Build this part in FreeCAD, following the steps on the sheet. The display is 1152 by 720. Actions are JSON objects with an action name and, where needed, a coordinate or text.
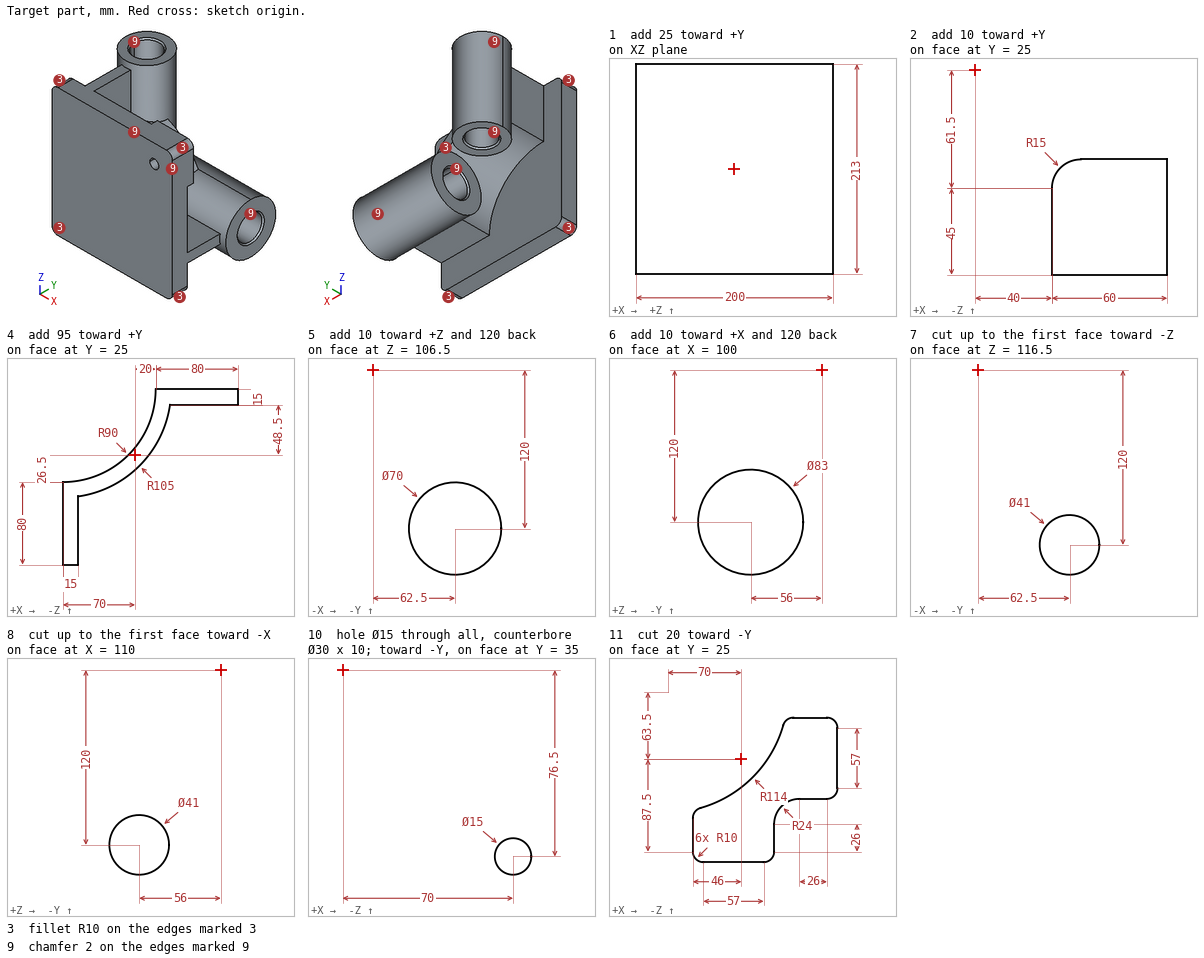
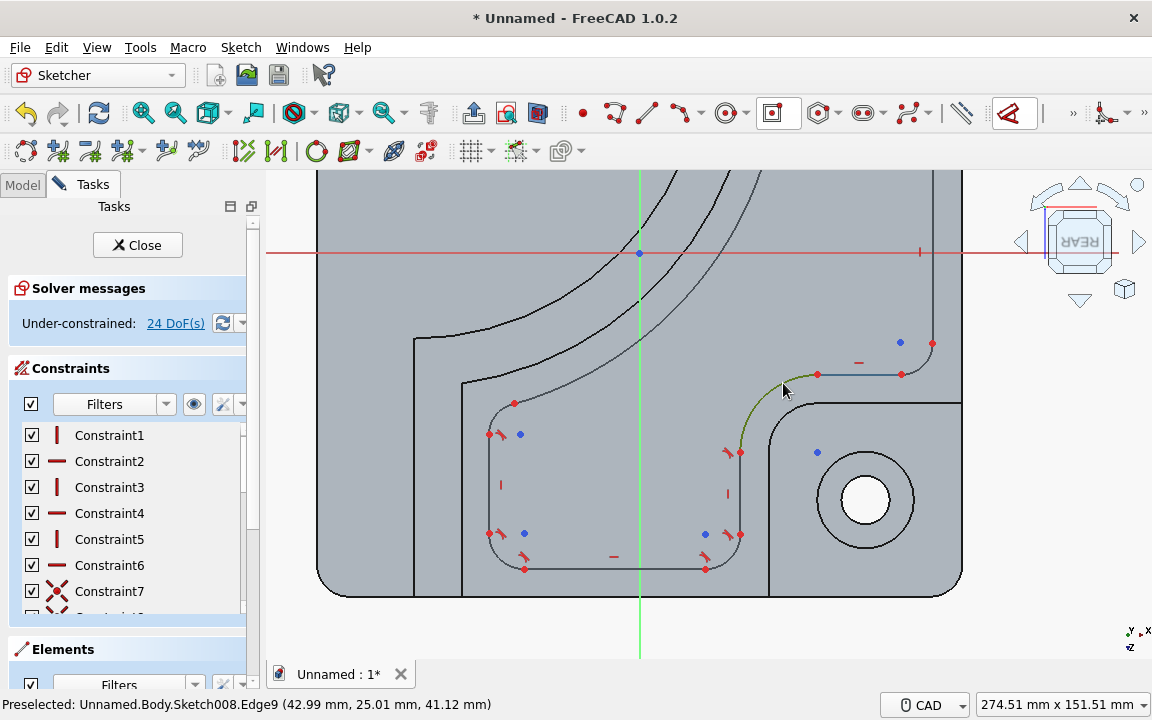
{"action": "key", "text": "t"}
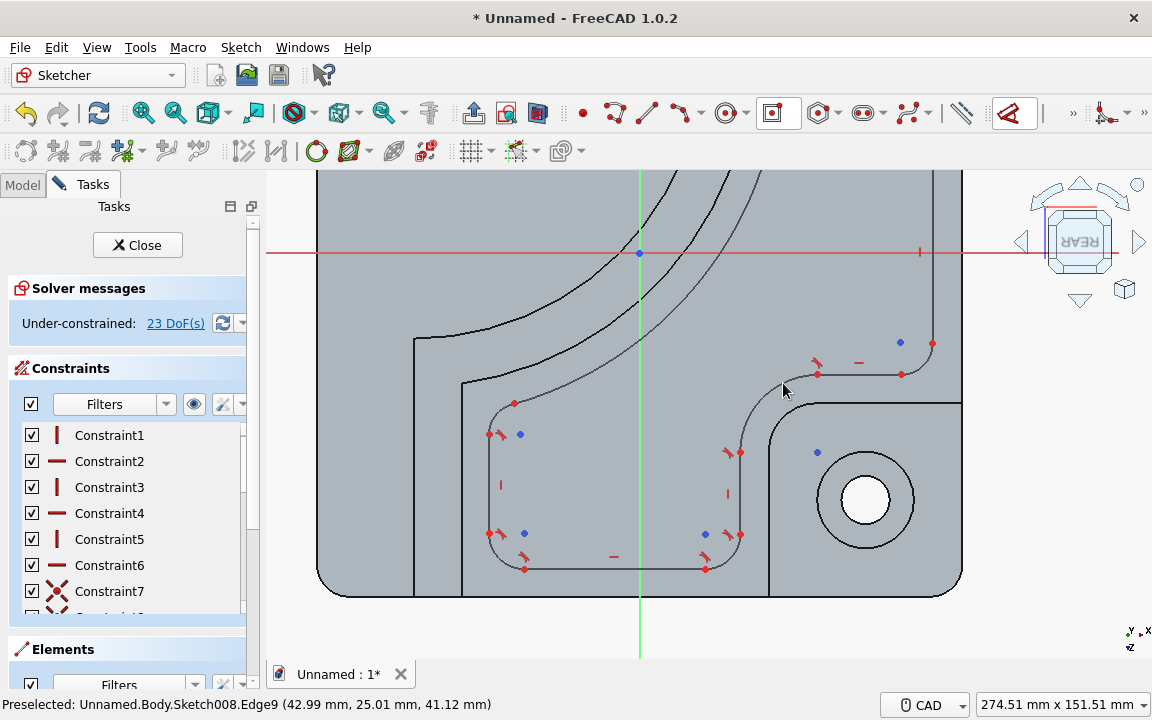
{"action": "left_click", "coordinate": [843, 375]}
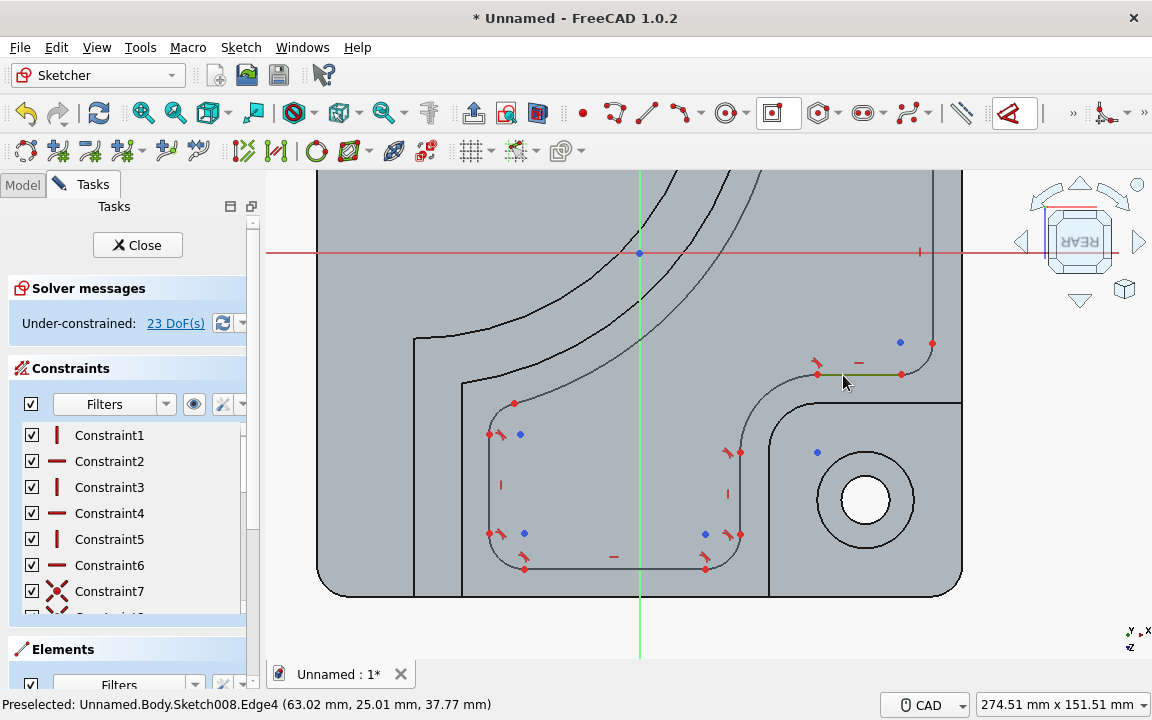
{"action": "left_click", "coordinate": [915, 371]}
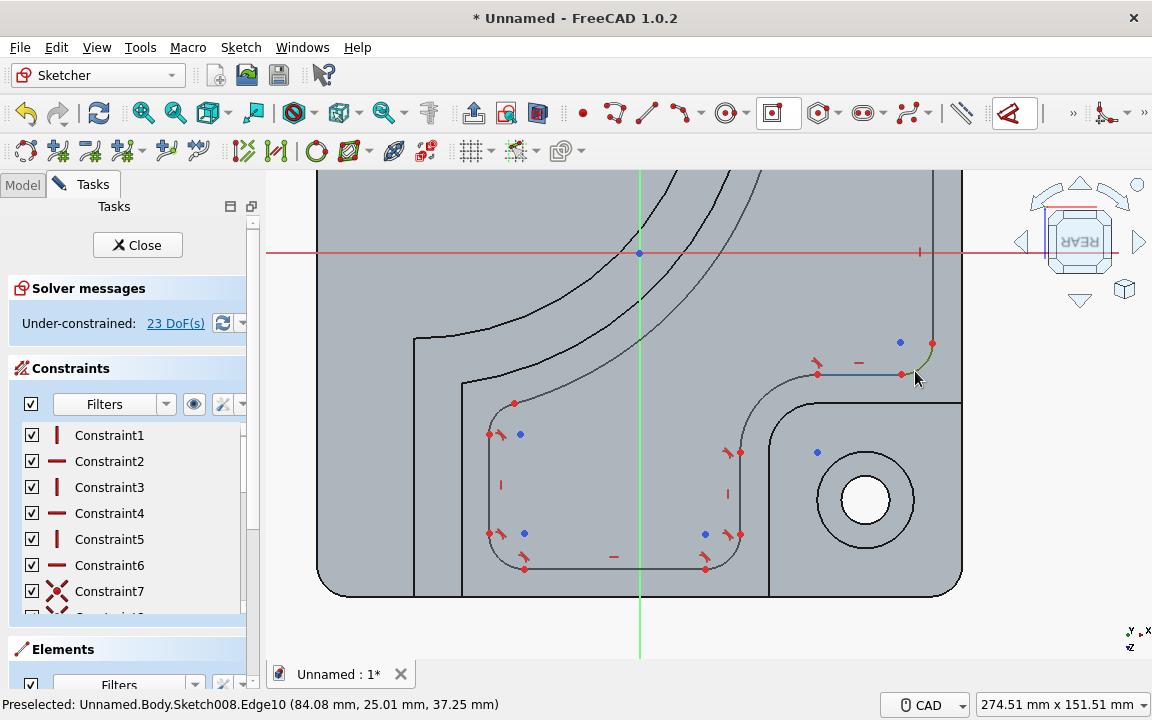
{"action": "key", "text": "t"}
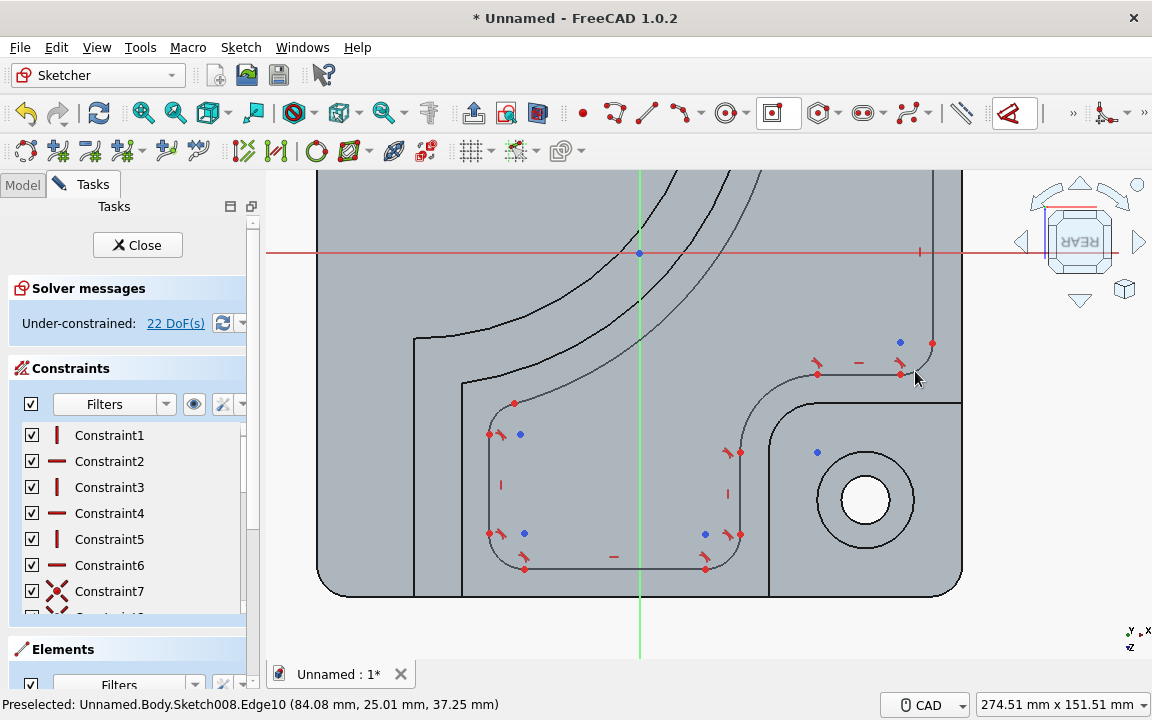
{"action": "left_click", "coordinate": [933, 288]}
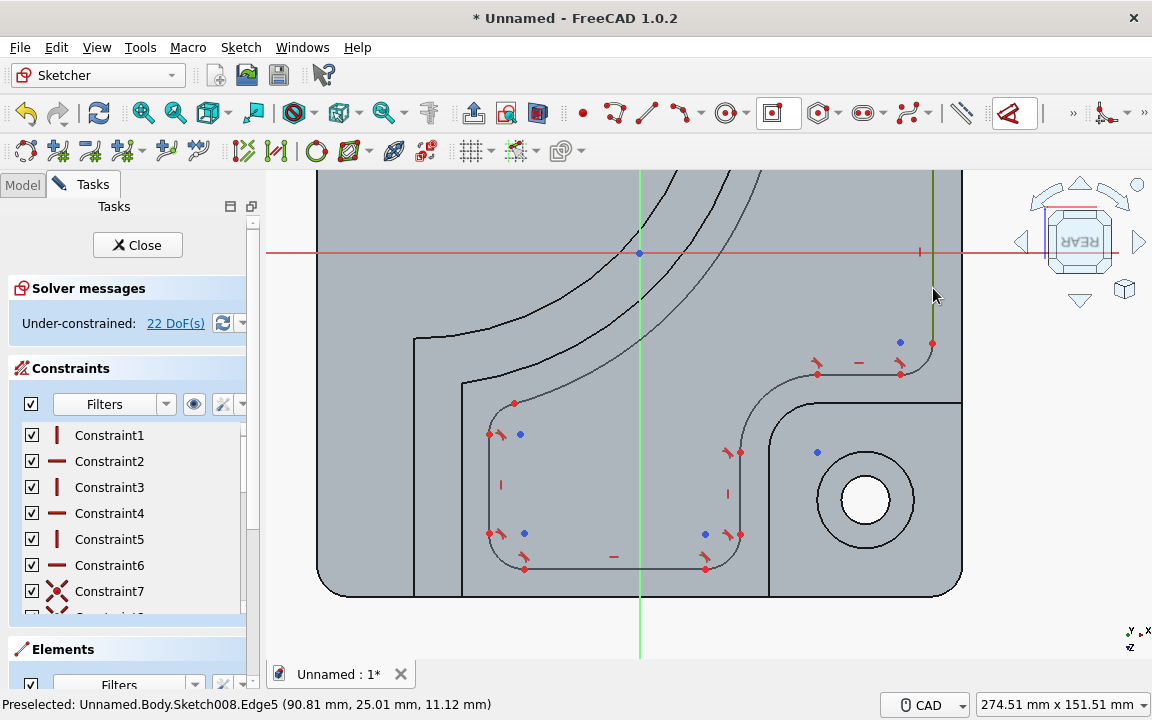
{"action": "left_click", "coordinate": [915, 372]}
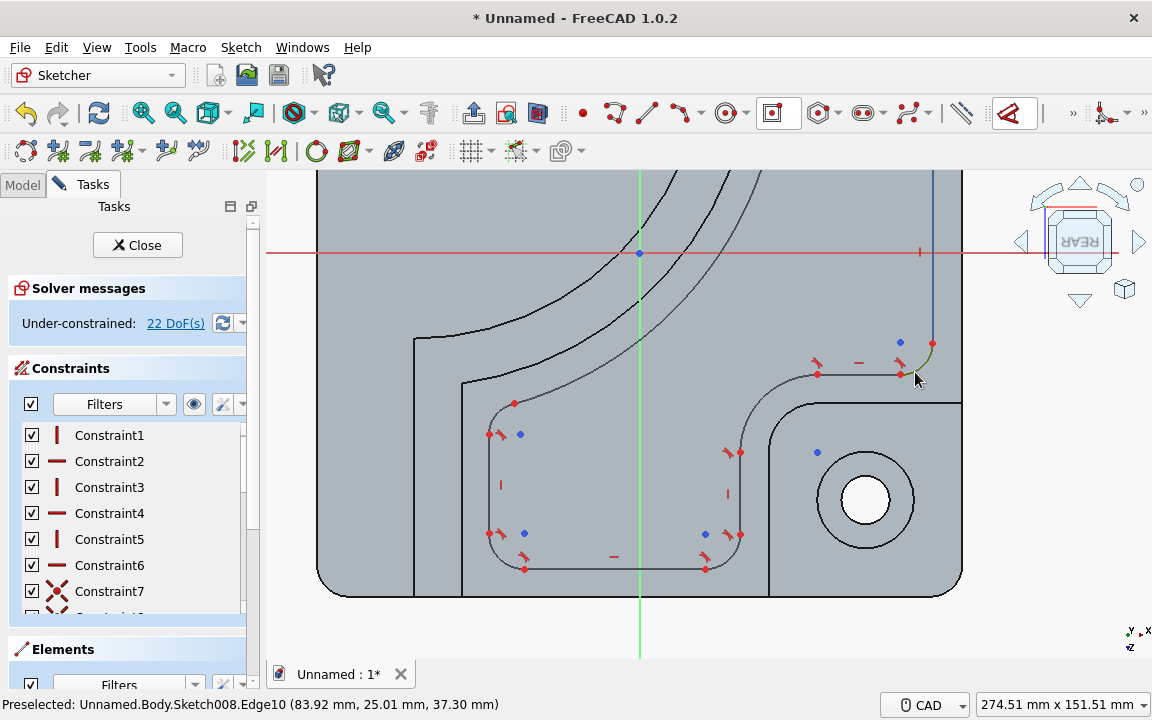
{"action": "key", "text": "t"}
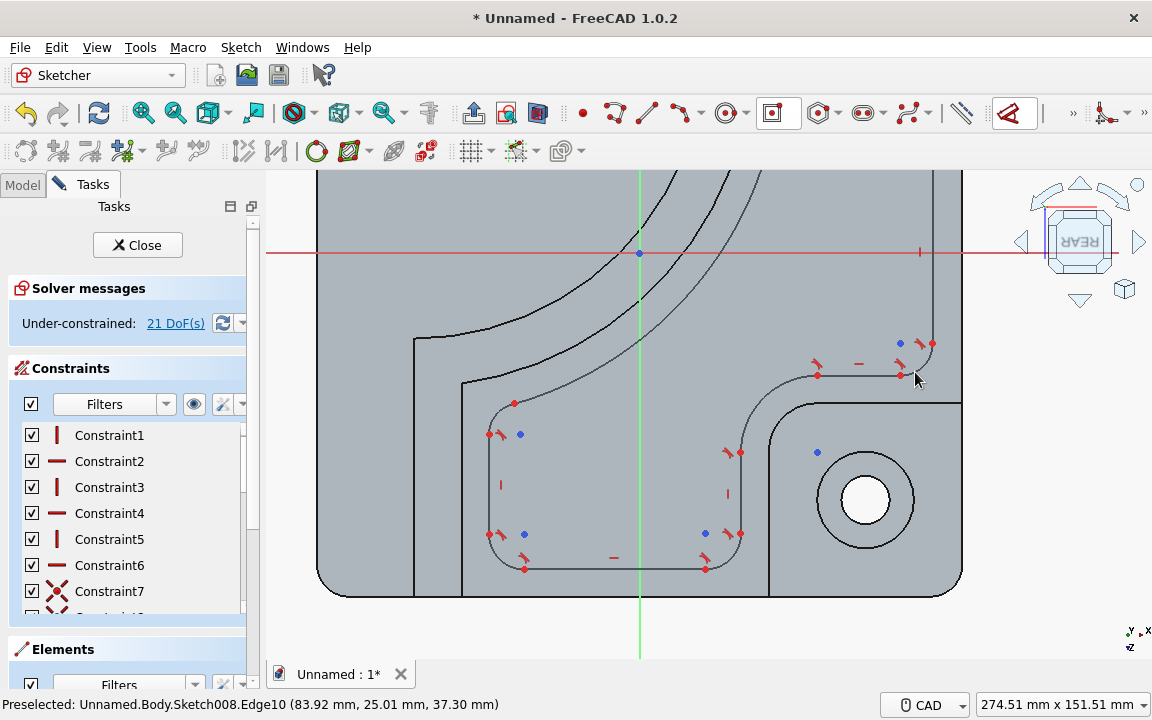
{"action": "left_click", "coordinate": [933, 288]}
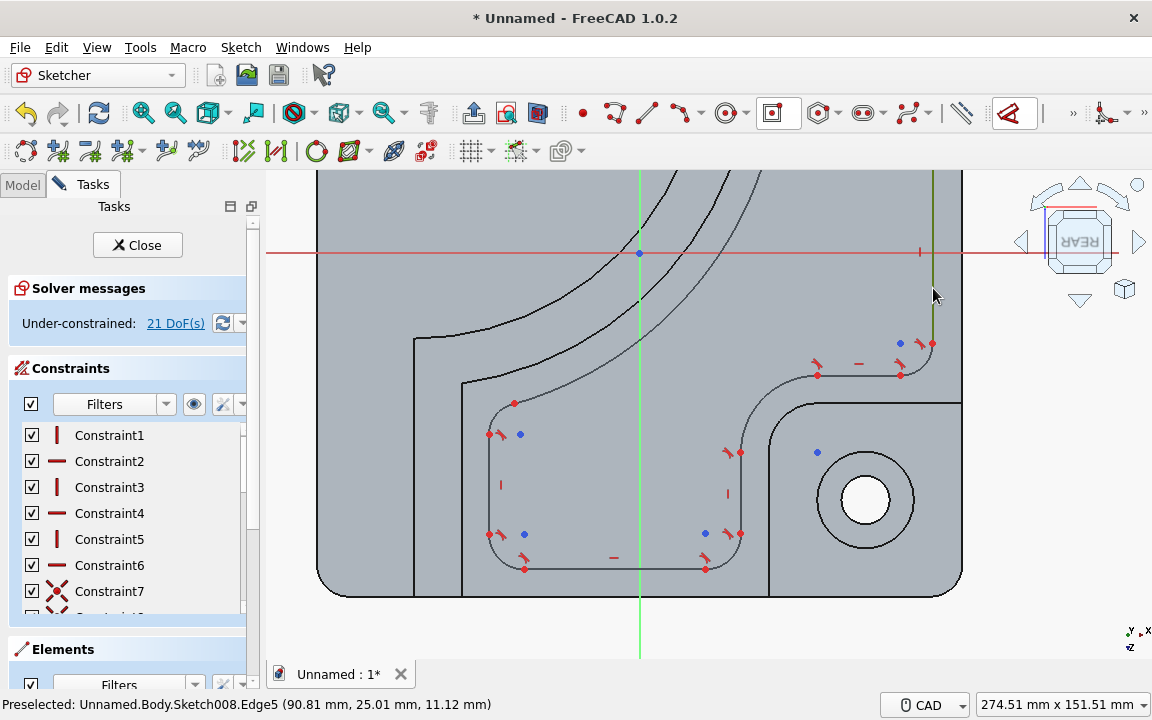
{"action": "scroll", "coordinate": [495, 552], "scroll_direction": "down", "scroll_amount": 2}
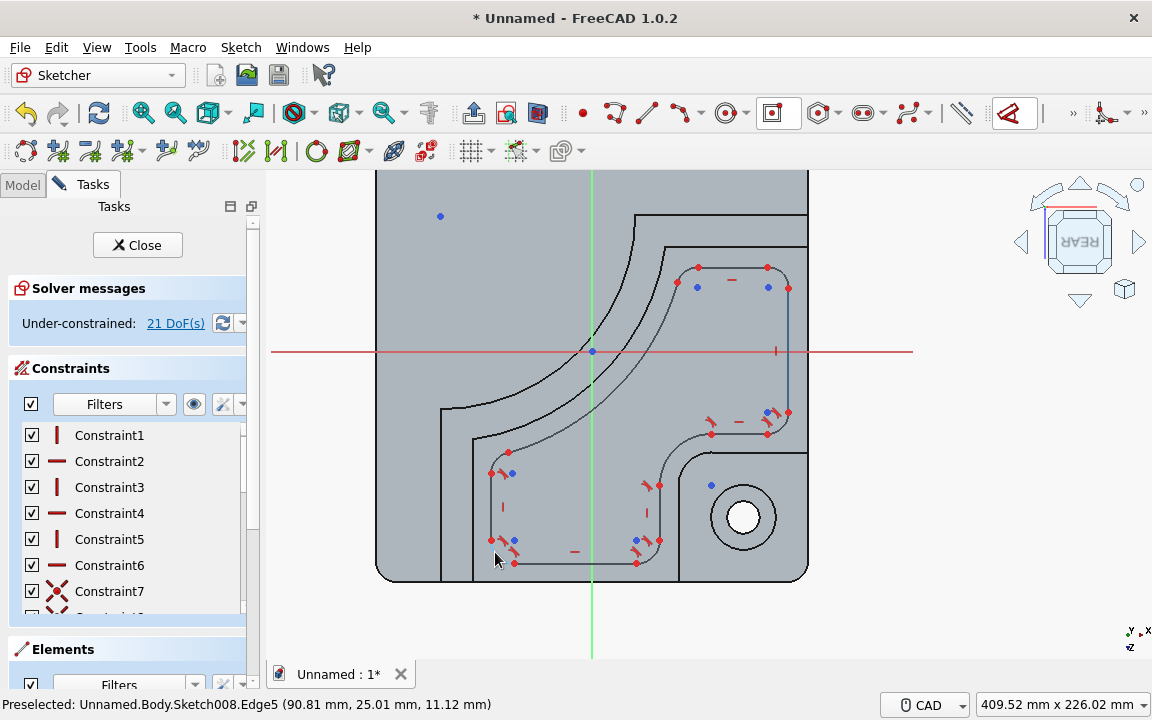
{"action": "scroll", "coordinate": [787, 279], "scroll_direction": "up", "scroll_amount": 2}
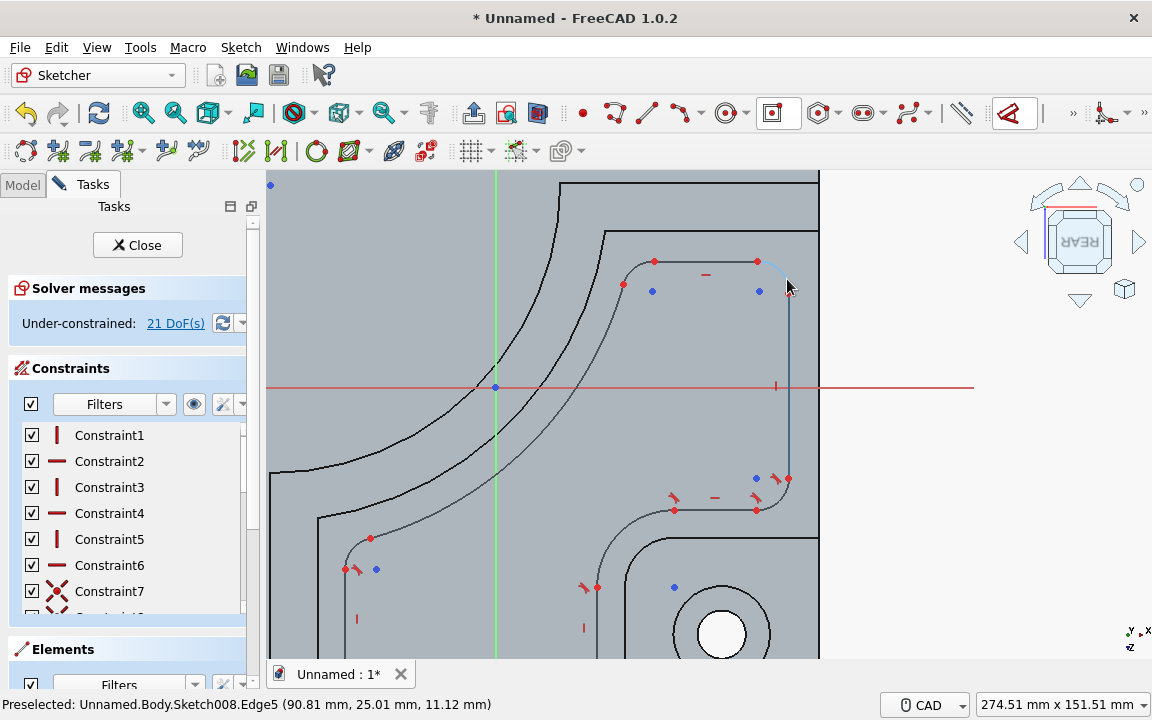
{"action": "left_click", "coordinate": [786, 279]}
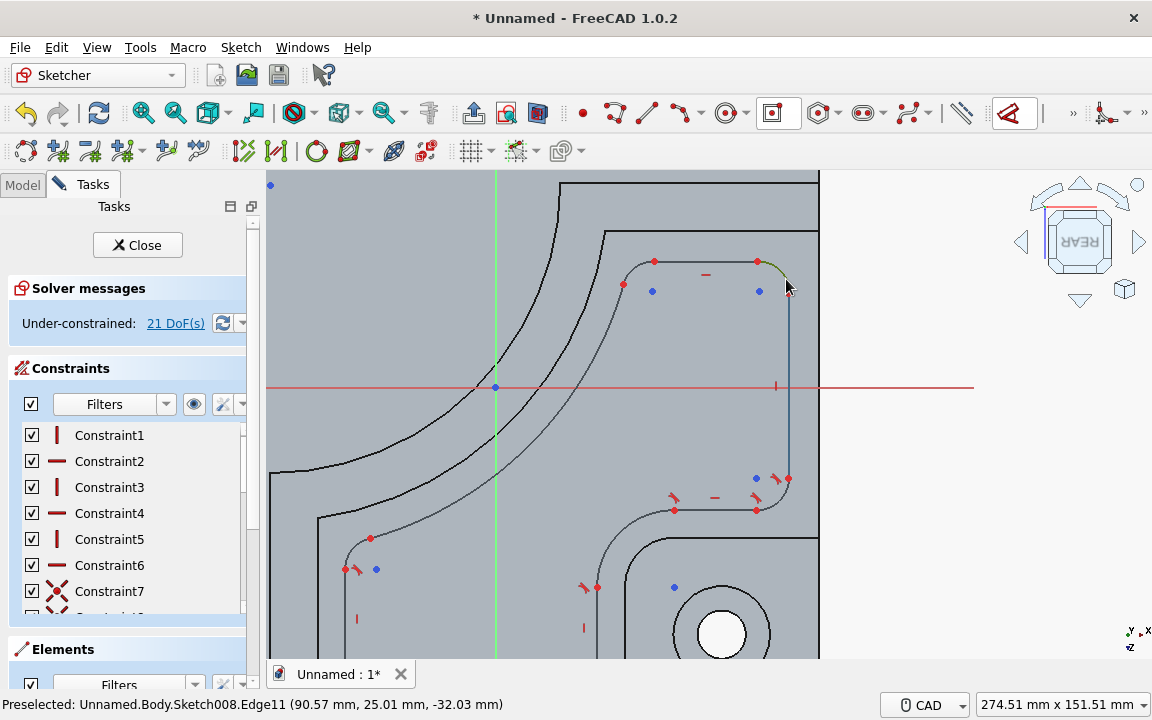
{"action": "key", "text": "t"}